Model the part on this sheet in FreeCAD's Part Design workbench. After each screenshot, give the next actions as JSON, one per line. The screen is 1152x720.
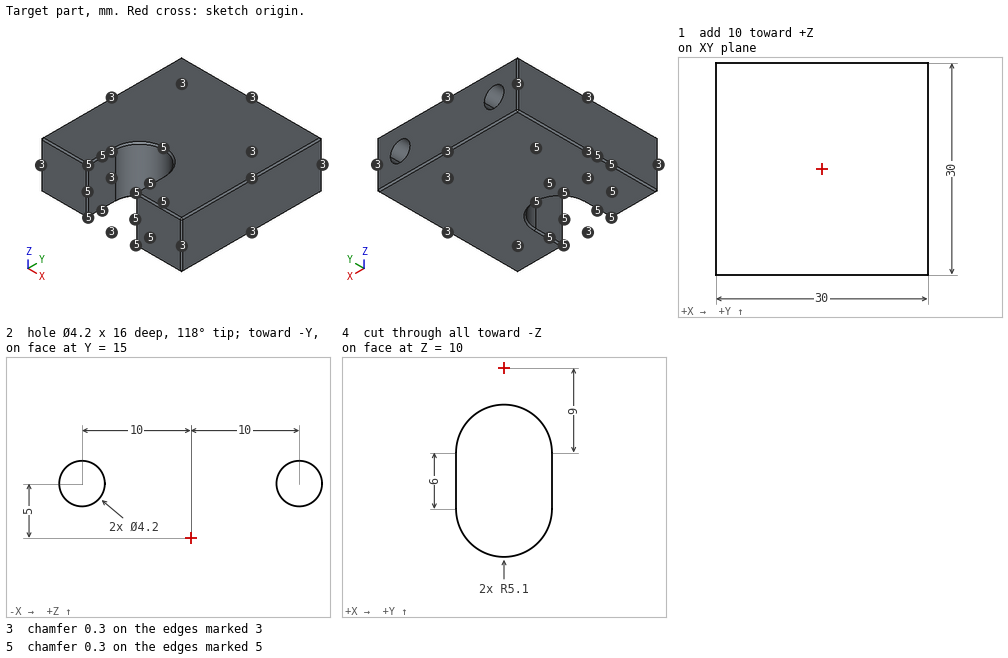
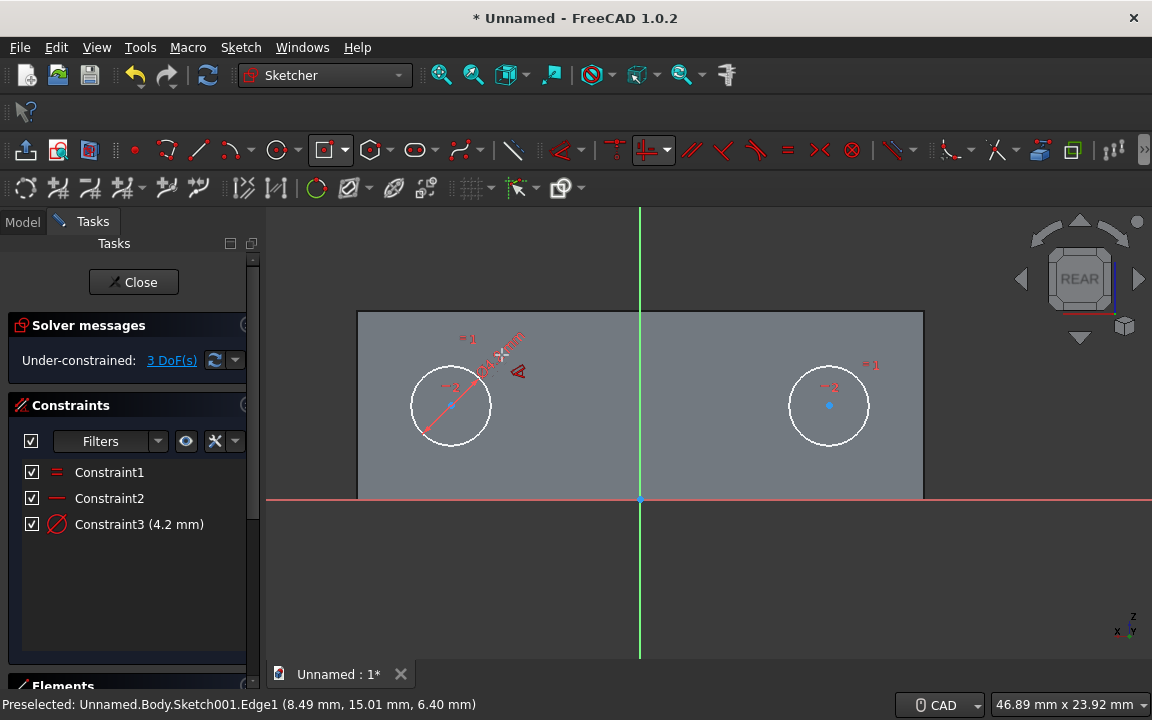
{"action": "left_click", "coordinate": [451, 406]}
{"action": "left_click", "coordinate": [417, 453]}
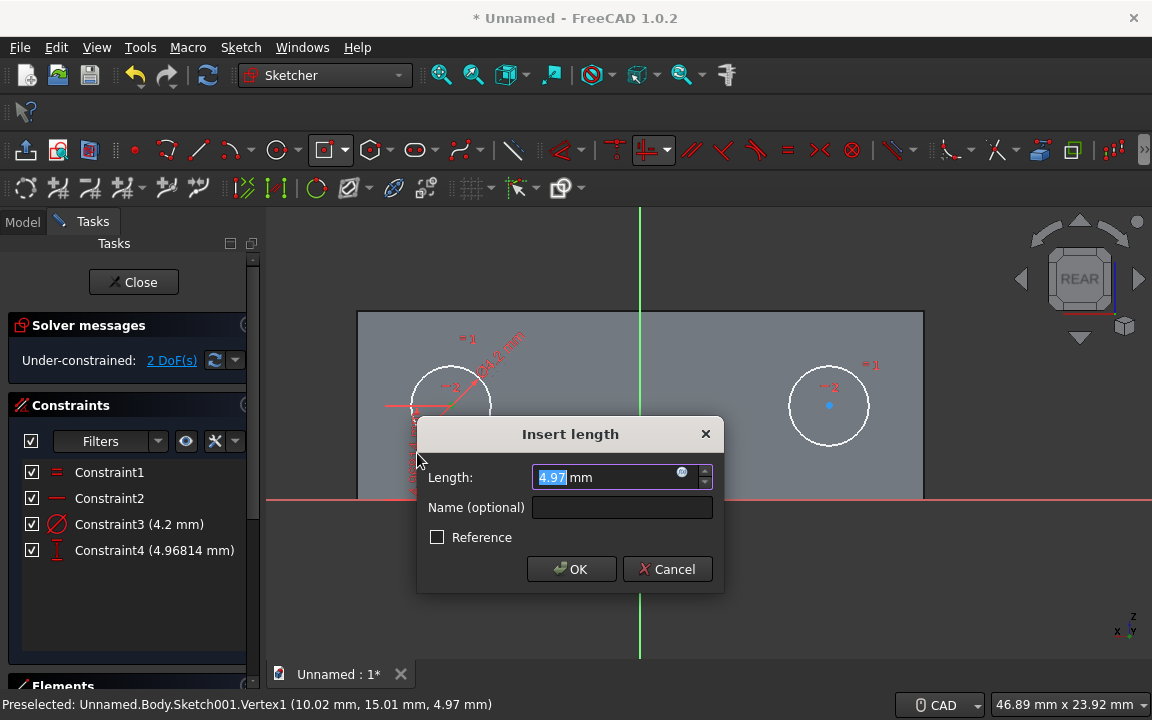
{"action": "type", "text": "5"}
{"action": "key", "text": "Return"}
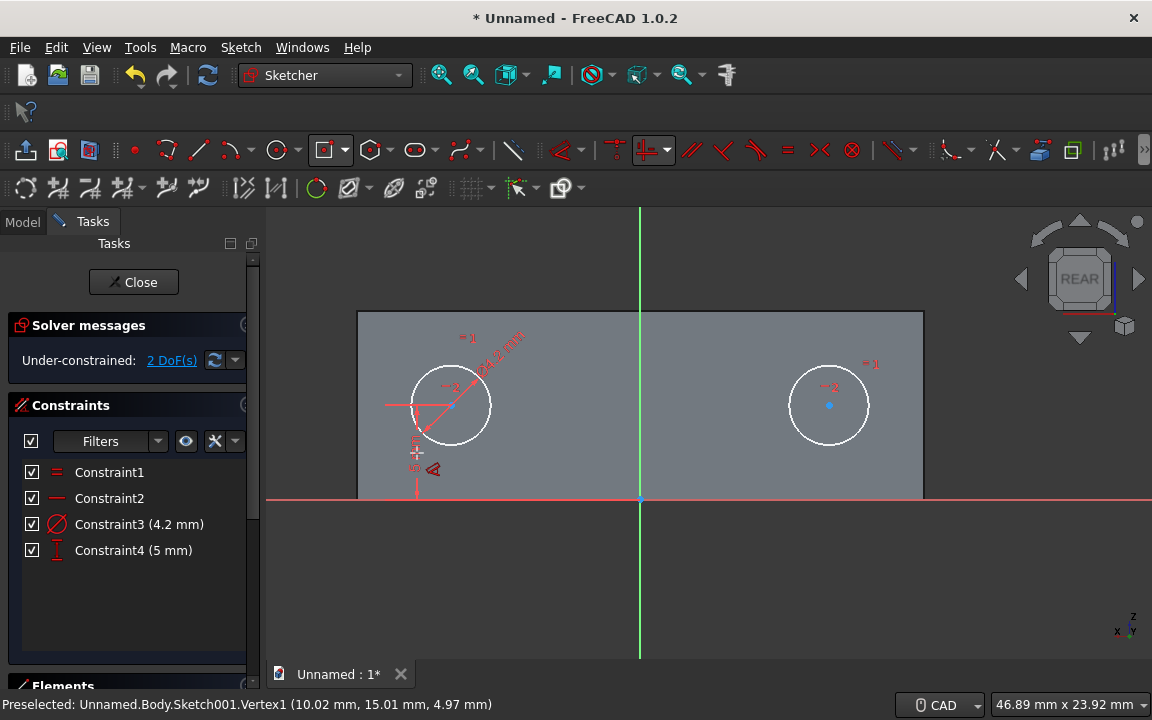
{"action": "left_click", "coordinate": [451, 405]}
{"action": "left_click", "coordinate": [546, 534]}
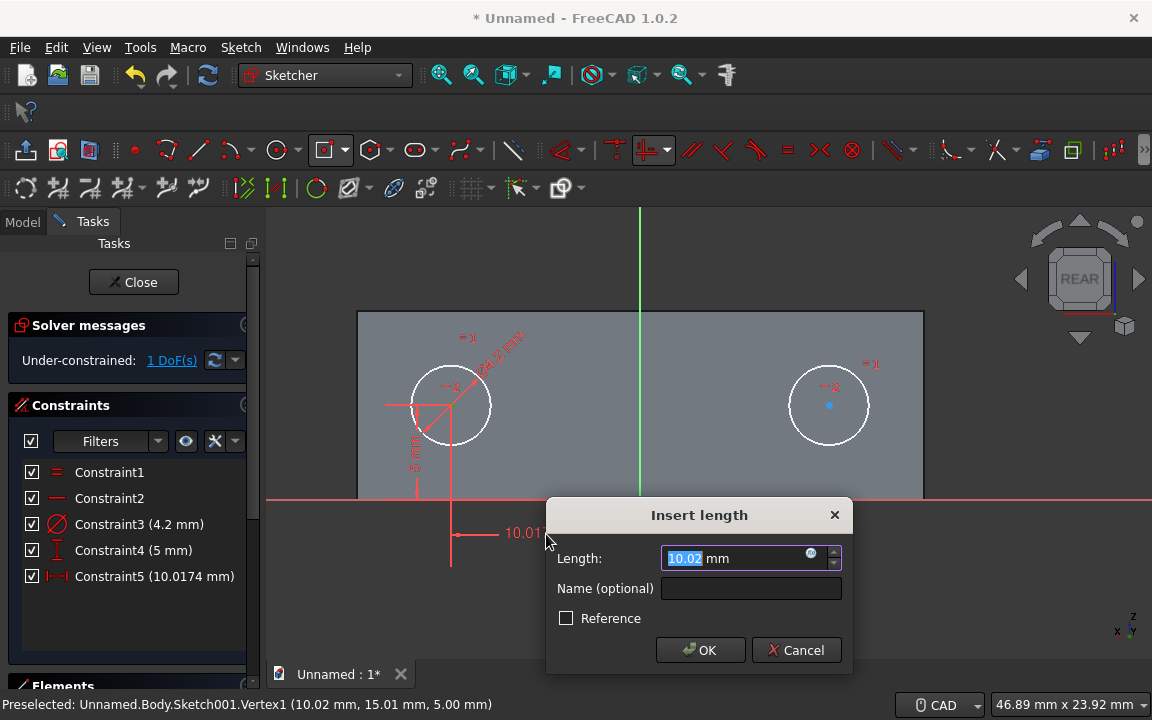
{"action": "type", "text": "10"}
{"action": "key", "text": "Return"}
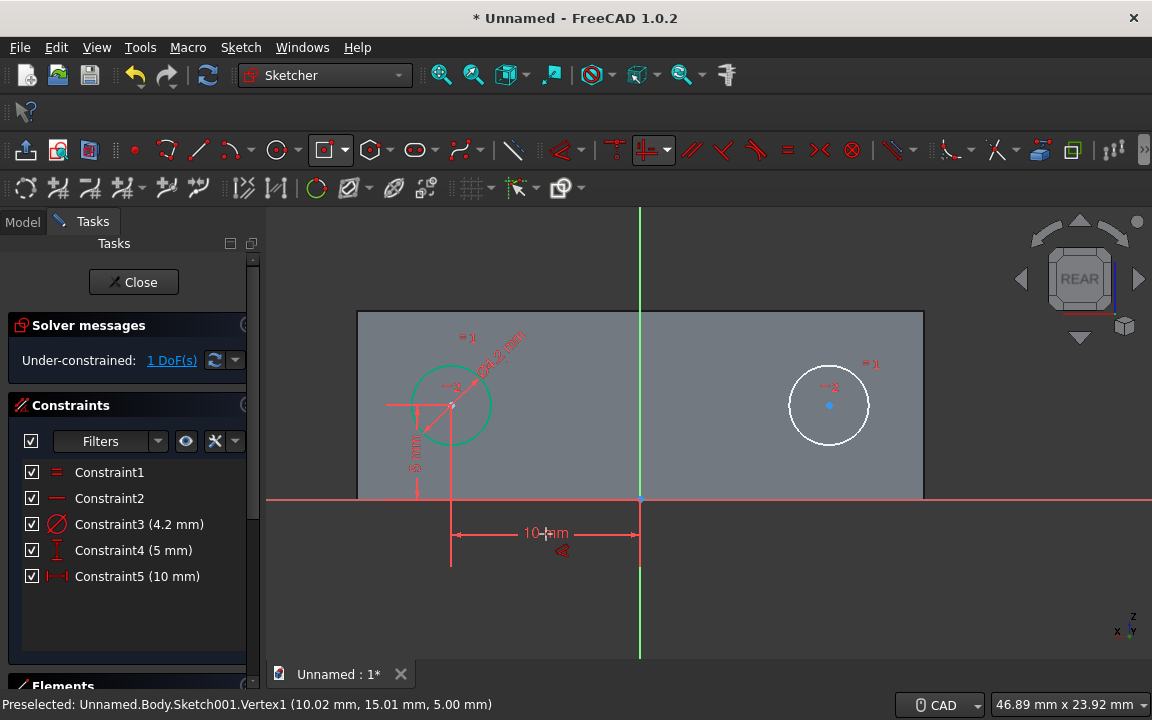
{"action": "left_click", "coordinate": [829, 405]}
{"action": "left_click", "coordinate": [735, 534]}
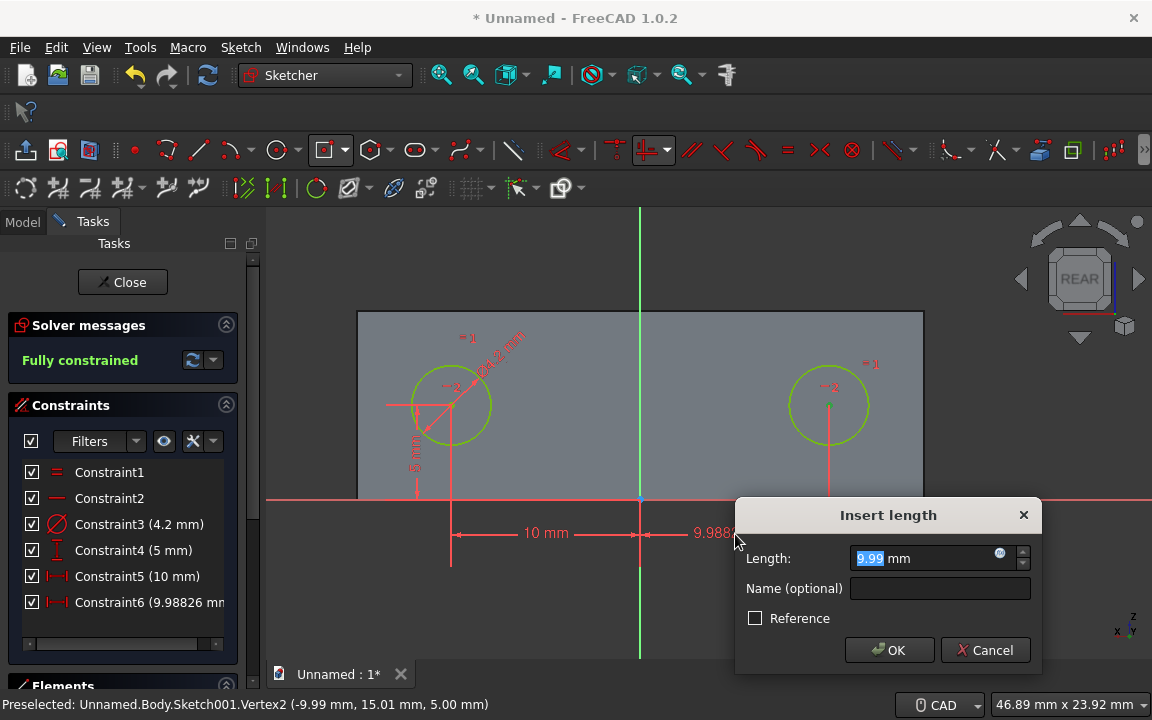
{"action": "type", "text": "10"}
{"action": "key", "text": "Return"}
{"action": "key", "text": "Escape"}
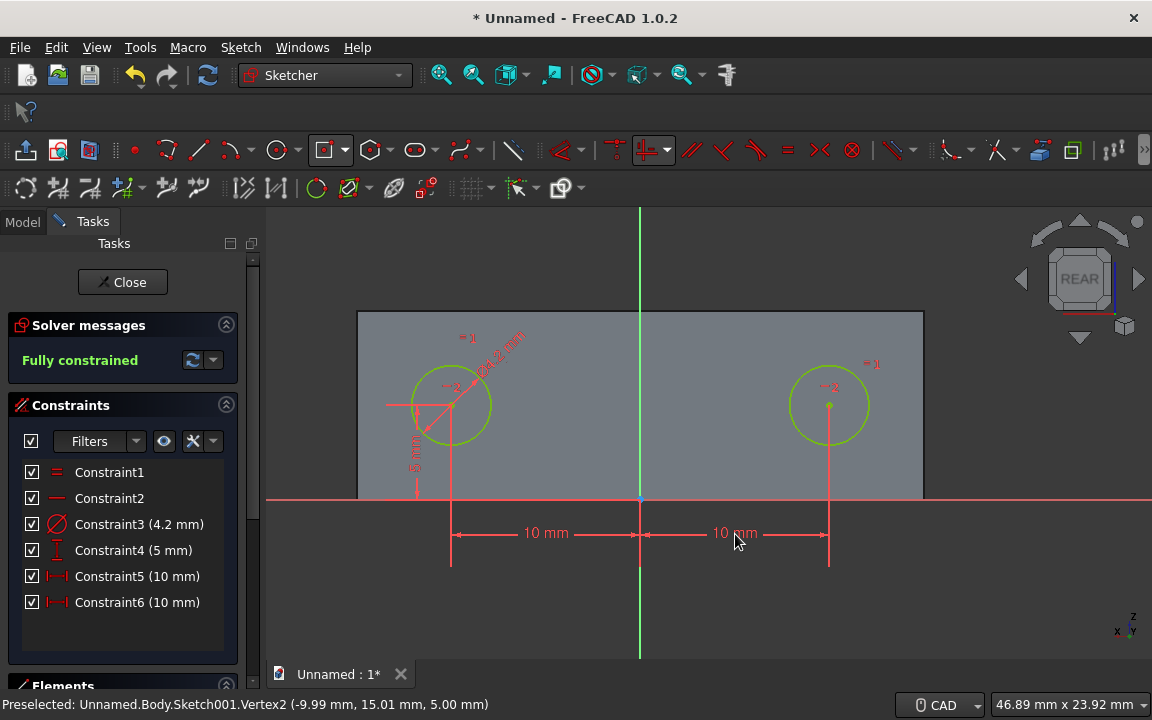
{"action": "left_click", "coordinate": [123, 282]}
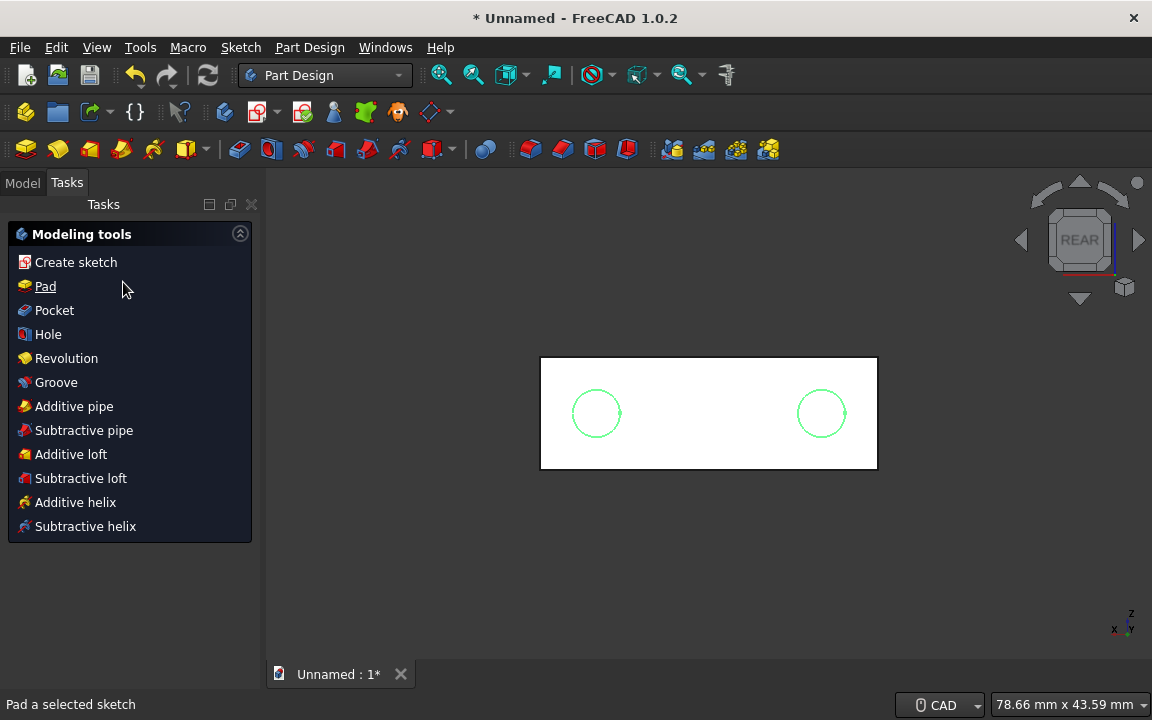
{"action": "left_click", "coordinate": [272, 150]}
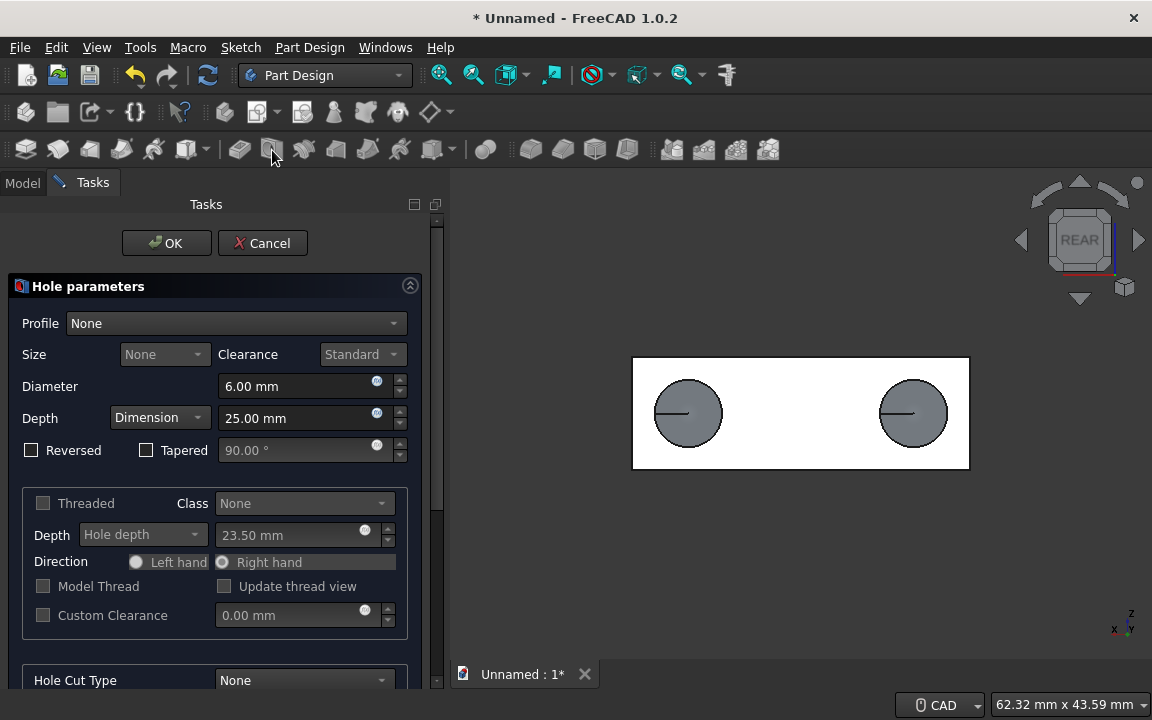
{"action": "triple_click", "coordinate": [305, 386]}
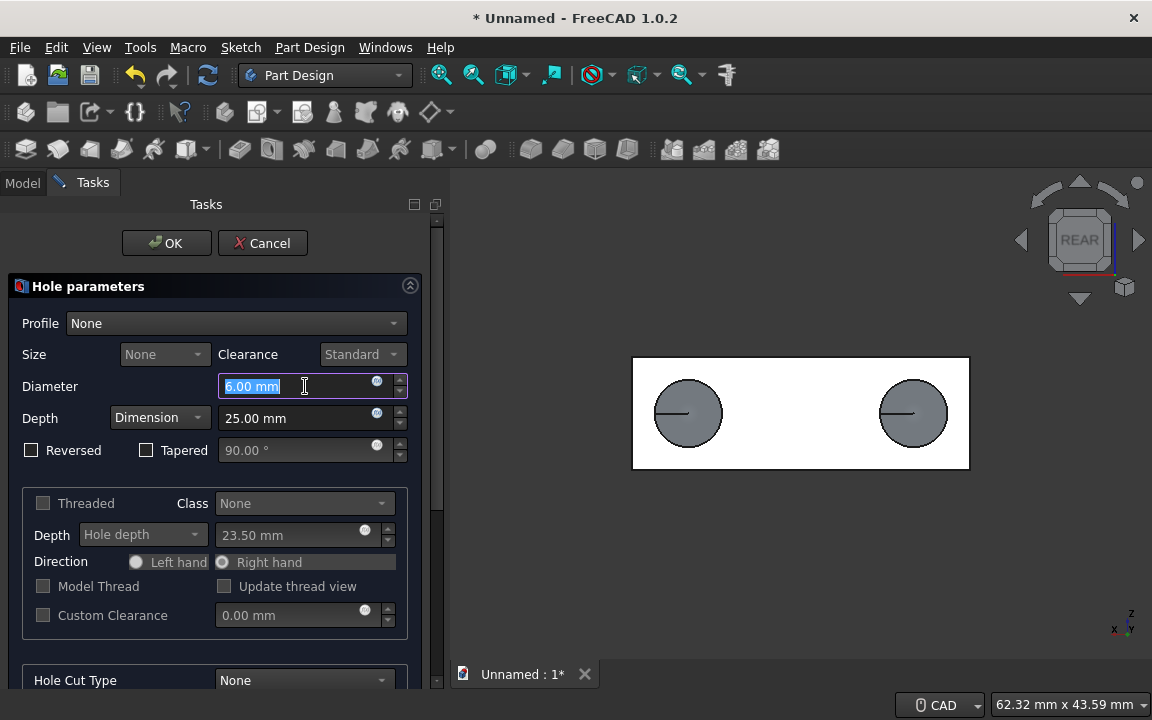
{"action": "type", "text": "4.2"}
{"action": "key", "text": "Tab"}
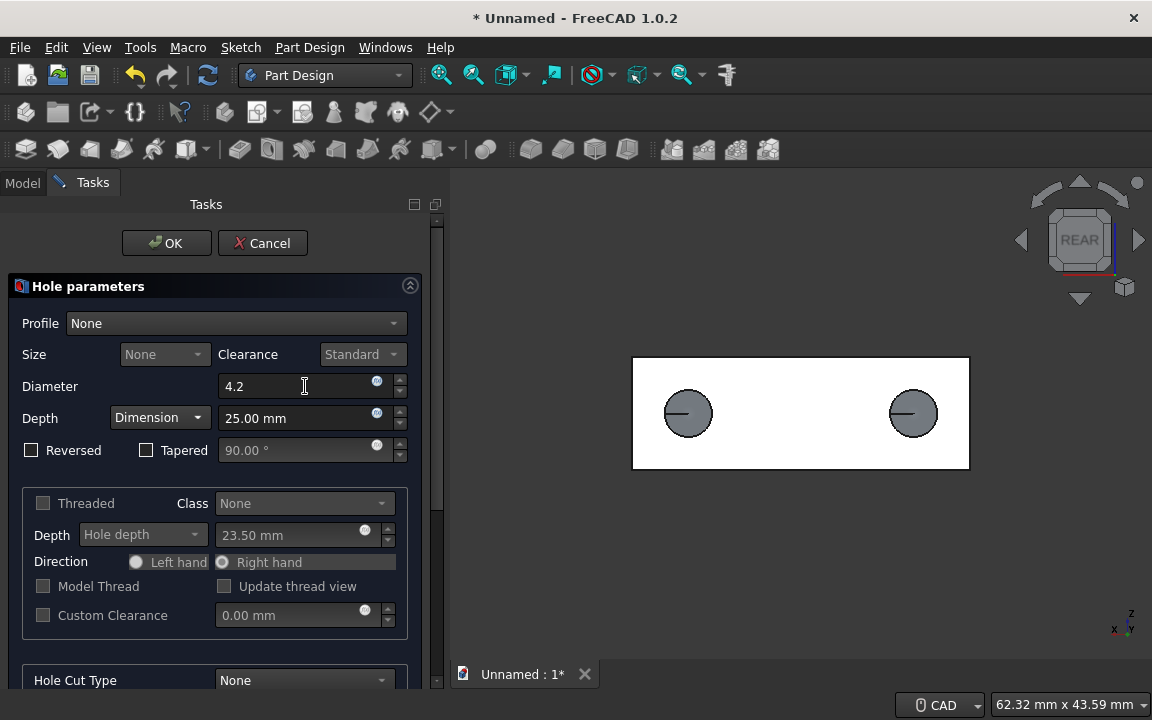
{"action": "triple_click", "coordinate": [305, 418]}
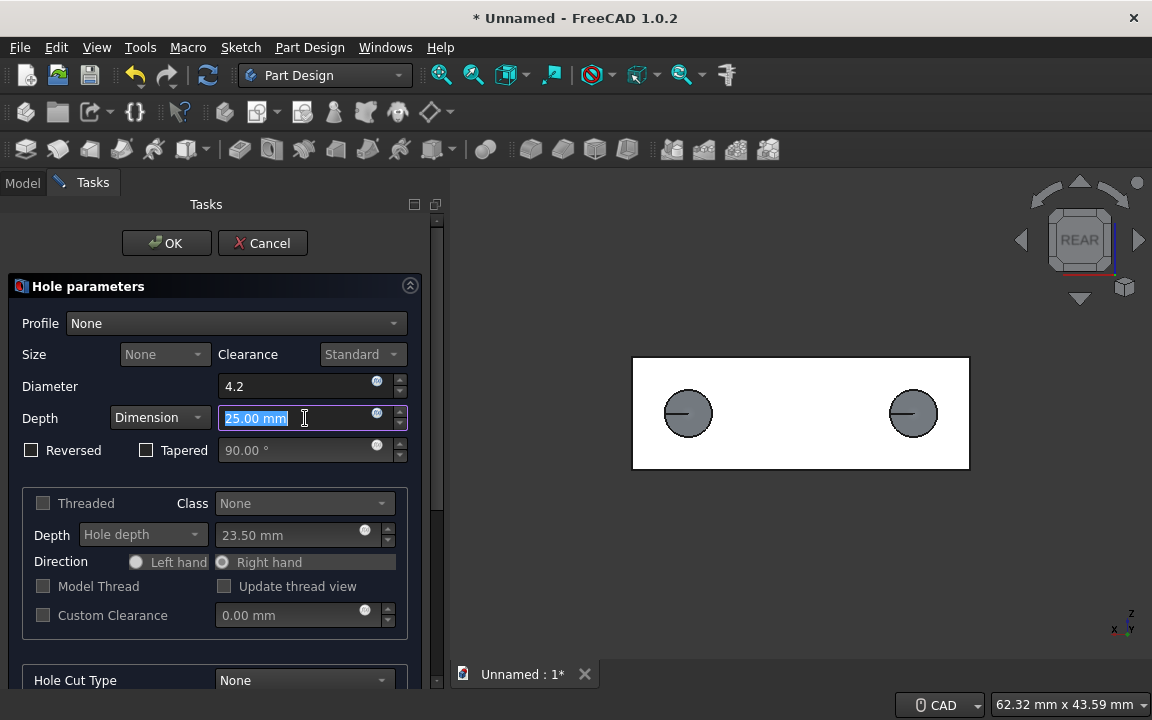
{"action": "type", "text": "16"}
{"action": "key", "text": "Tab"}